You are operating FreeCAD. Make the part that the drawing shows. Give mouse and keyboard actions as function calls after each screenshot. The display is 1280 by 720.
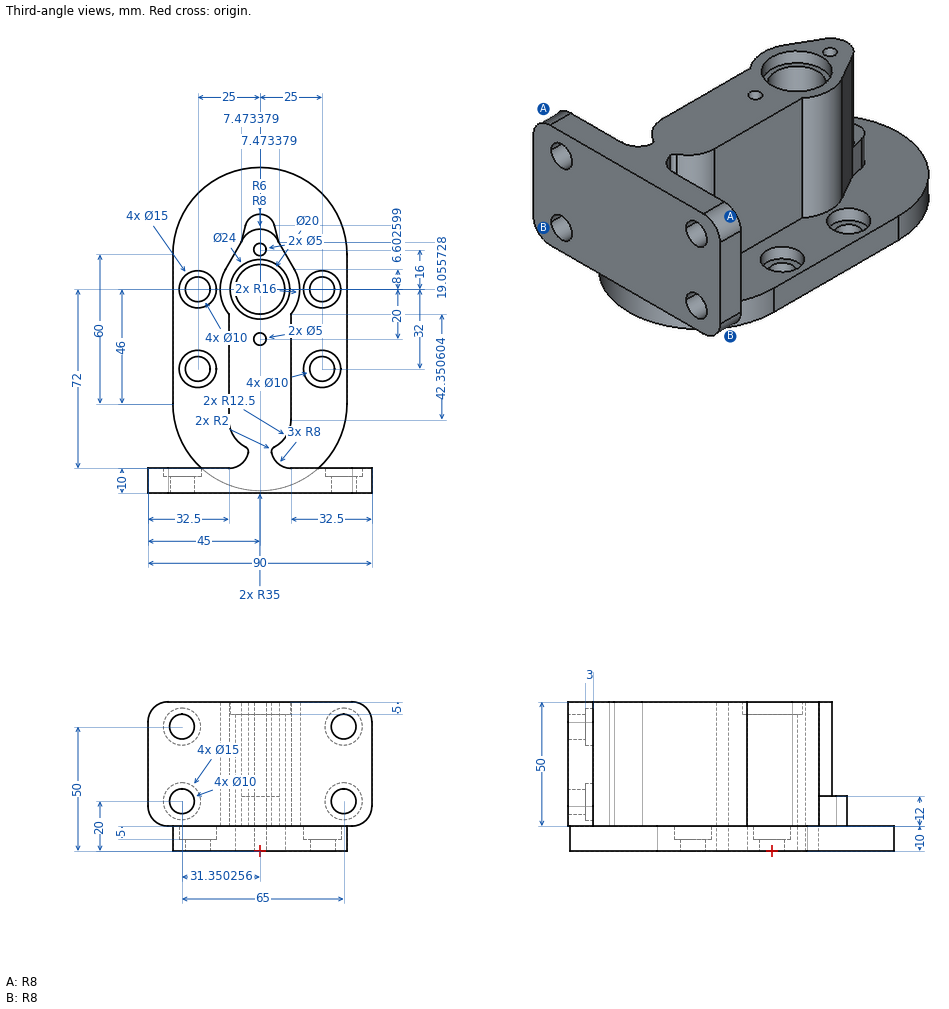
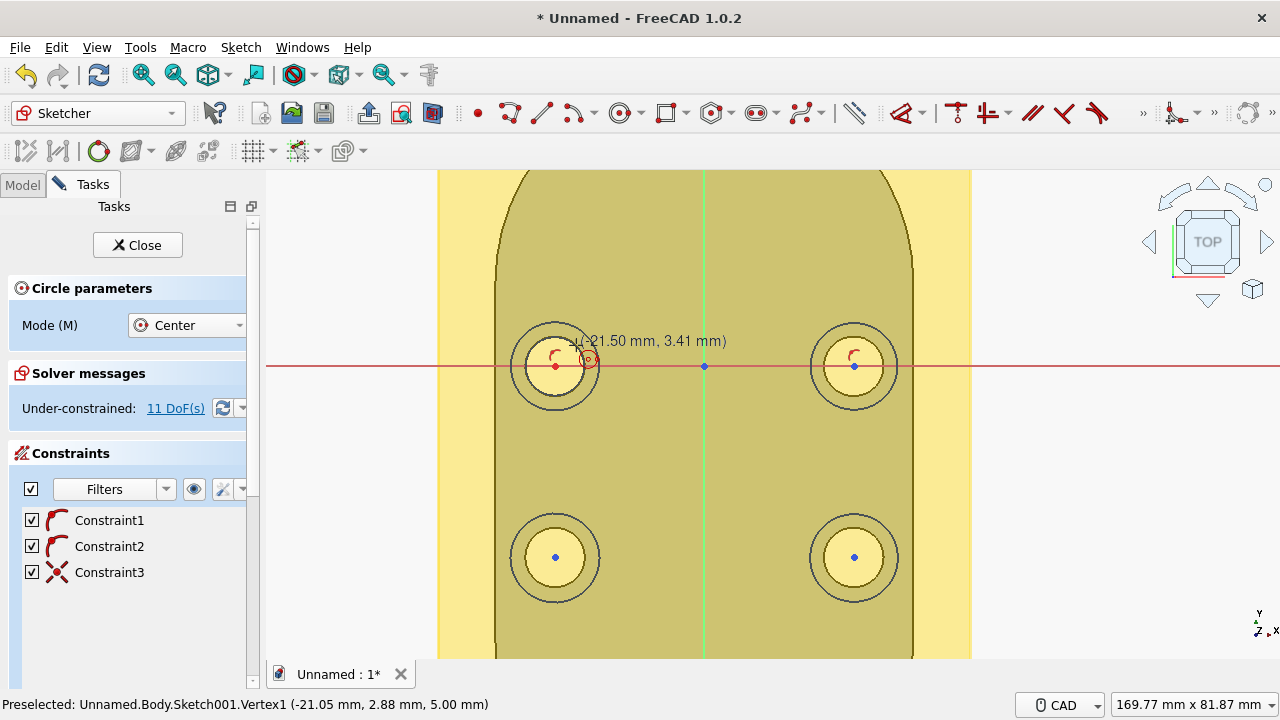
click(854, 366)
click(875, 345)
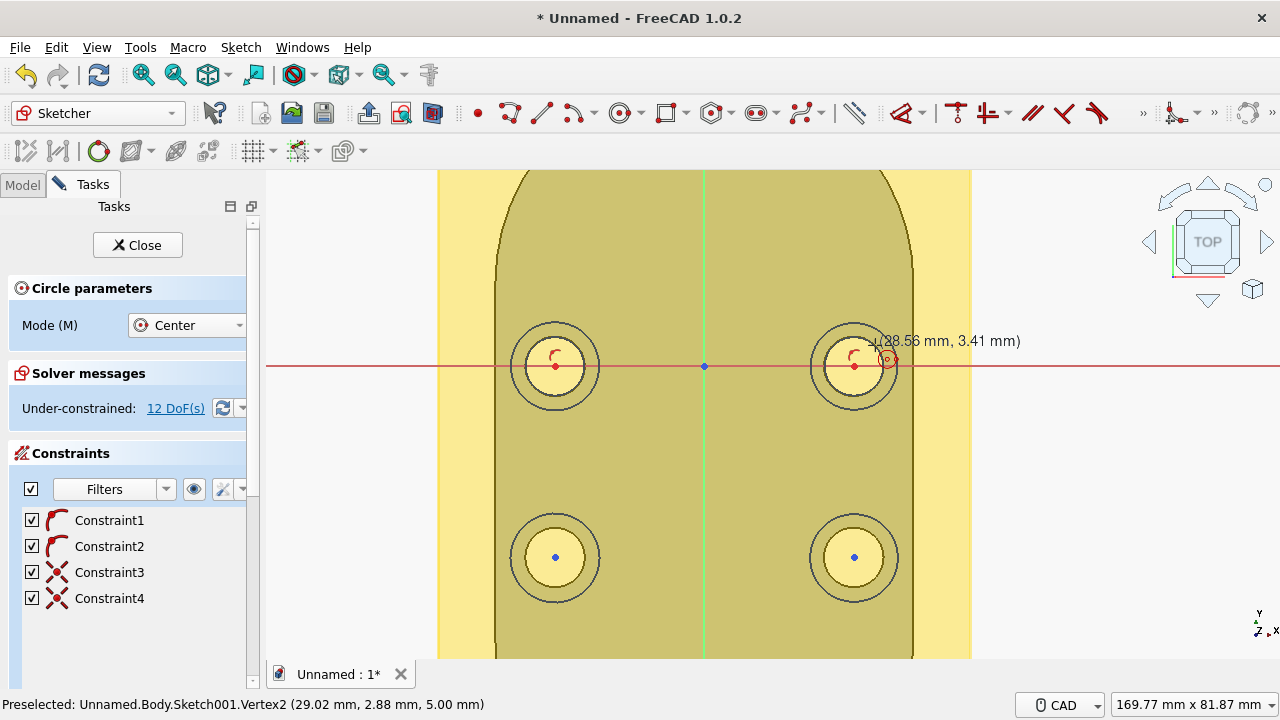
click(854, 558)
click(875, 536)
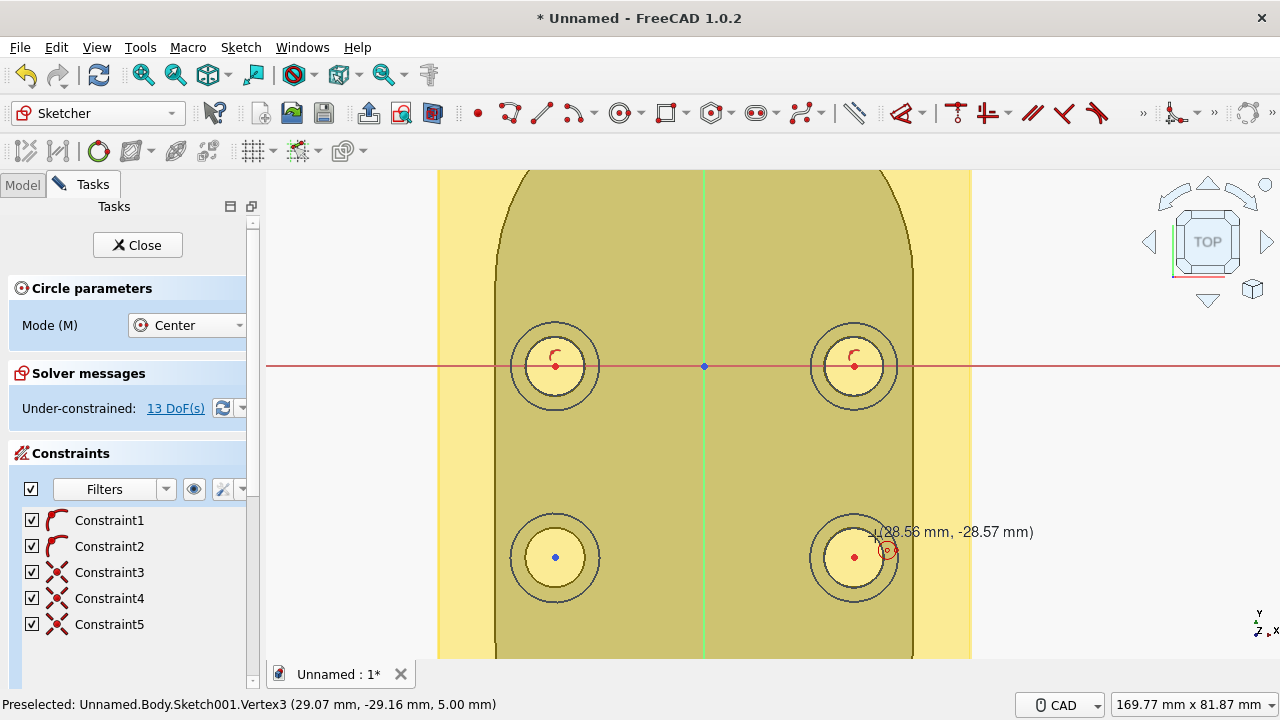
click(555, 558)
click(576, 536)
key(Escape)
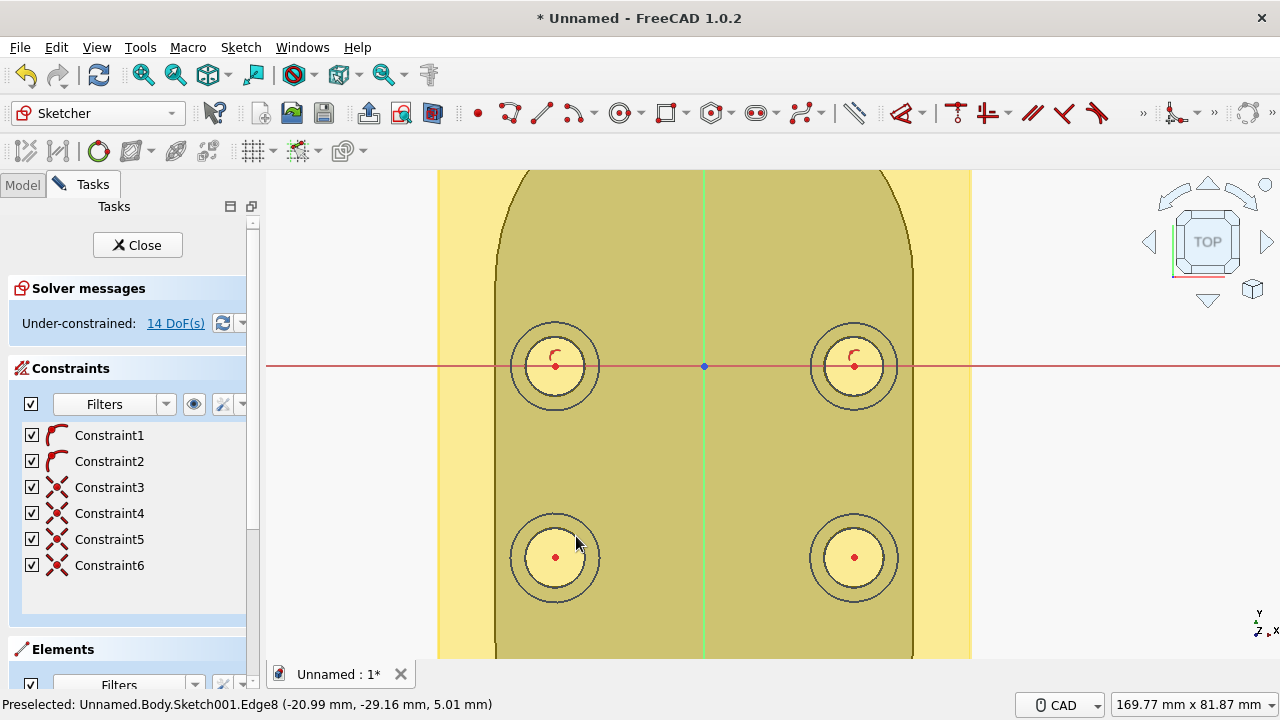
click(586, 335)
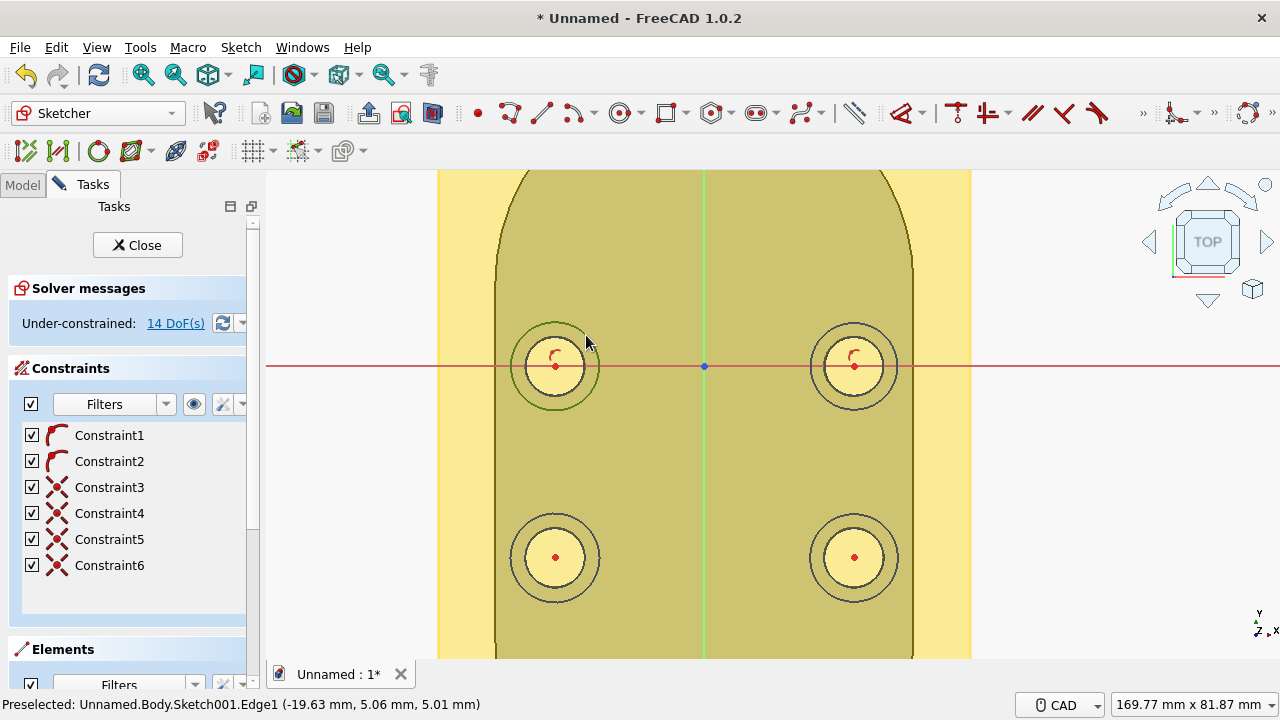
click(885, 336)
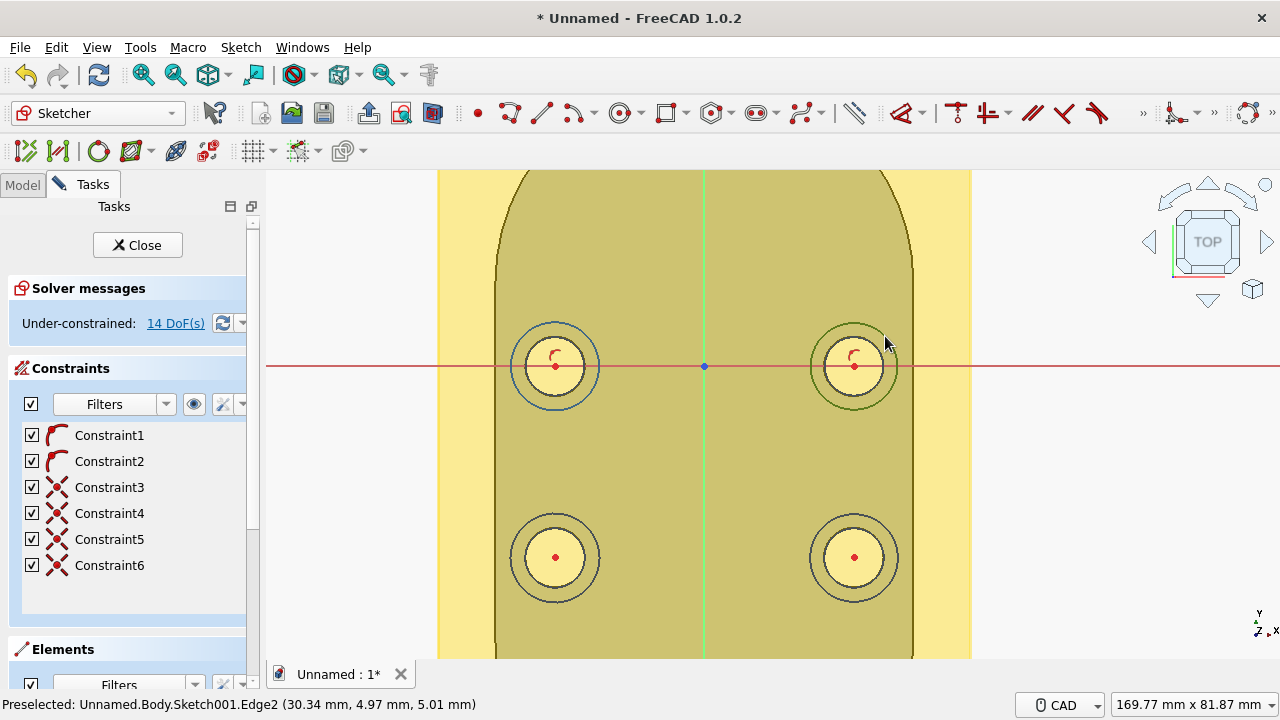
click(885, 527)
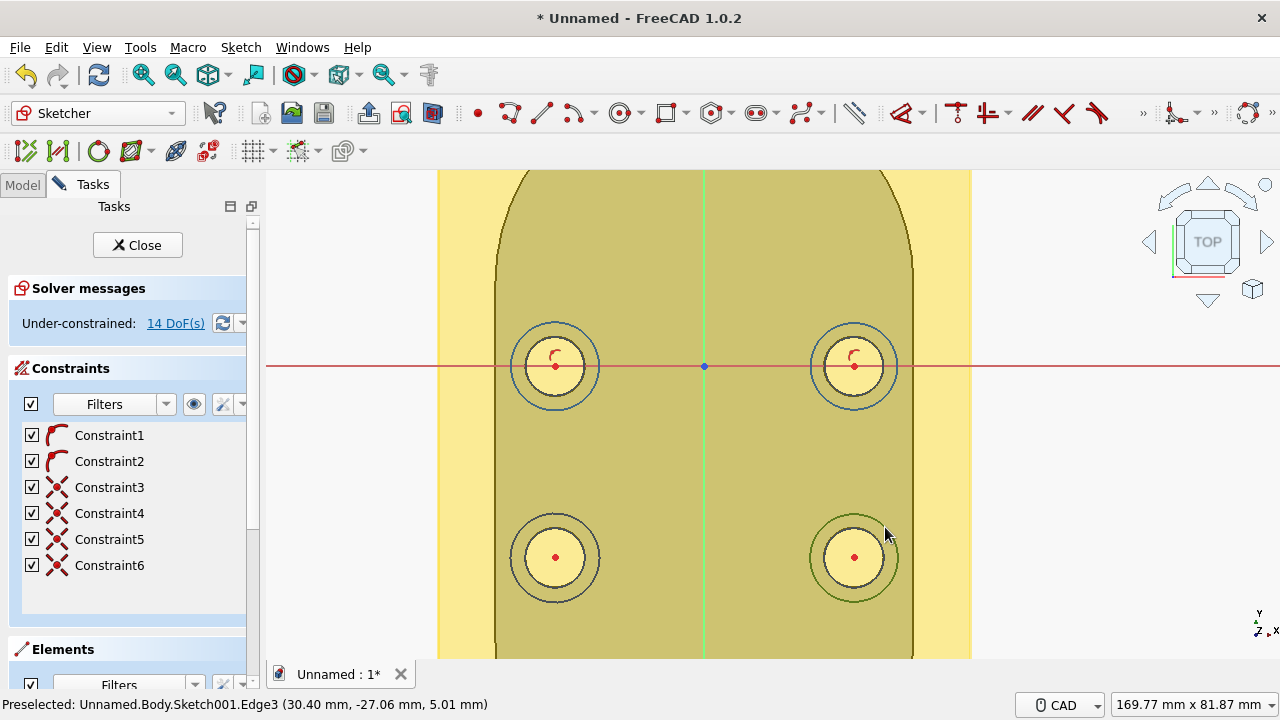
click(586, 526)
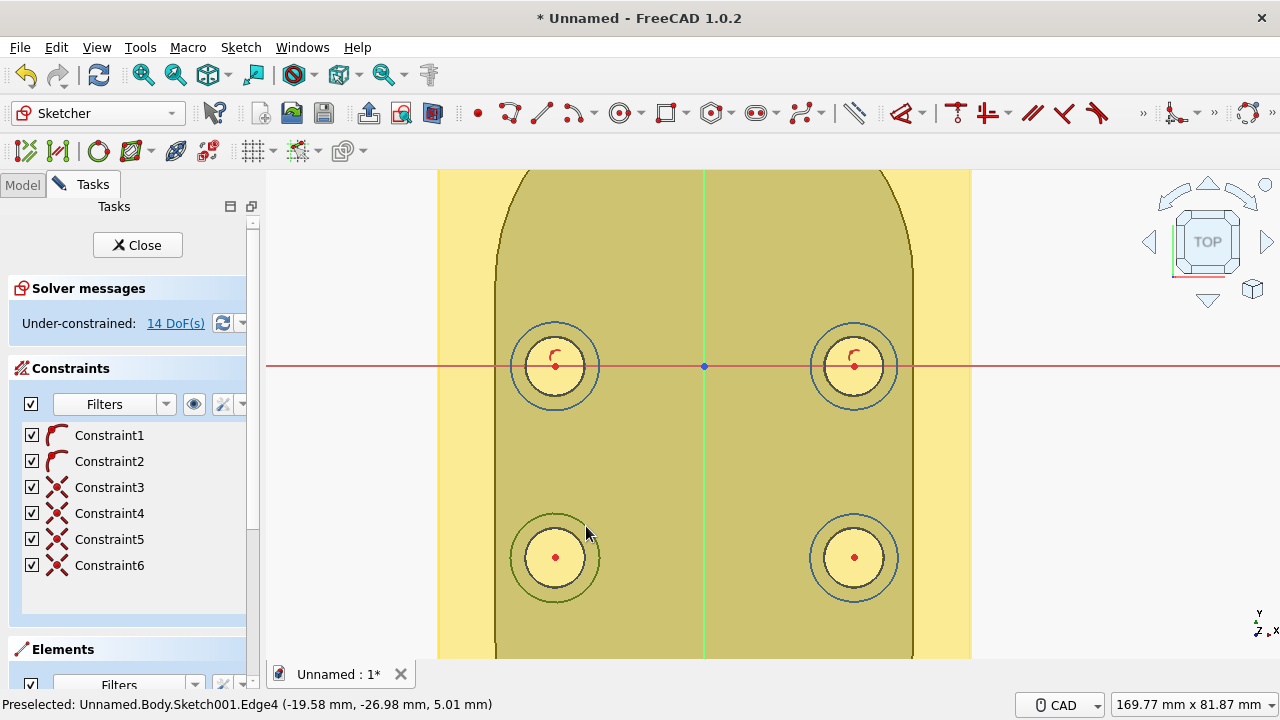
key(e)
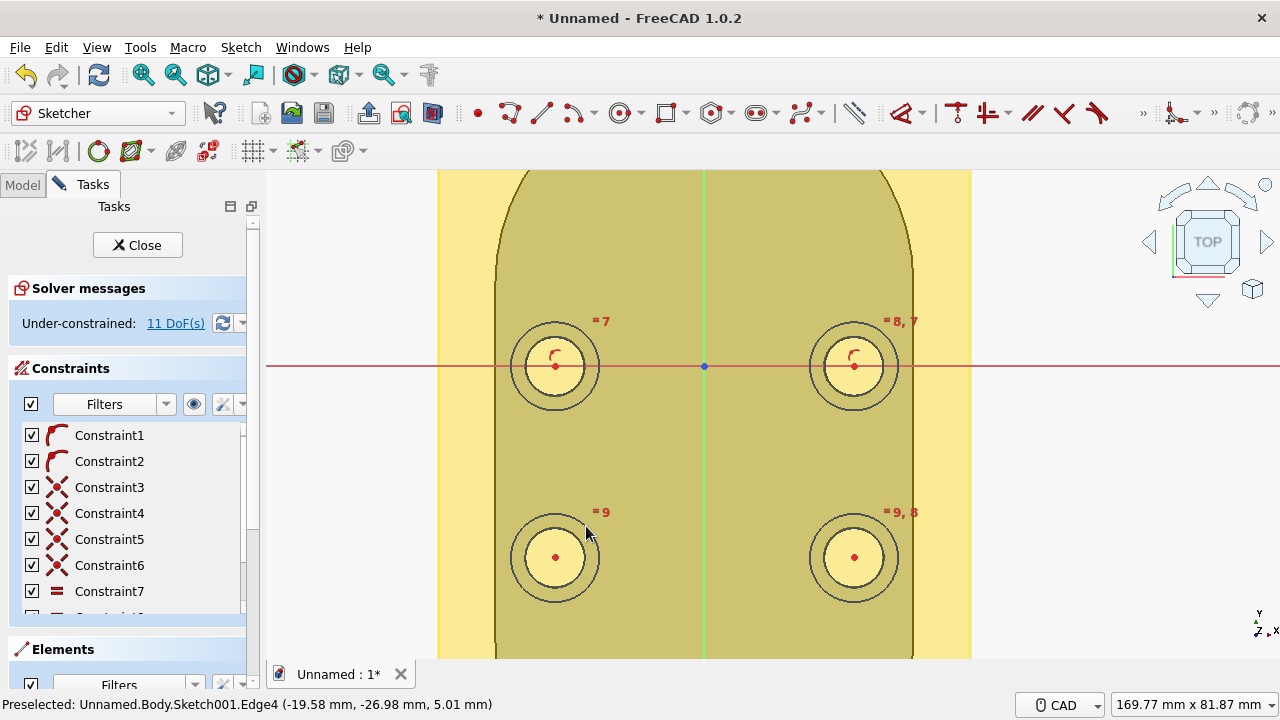
click(576, 346)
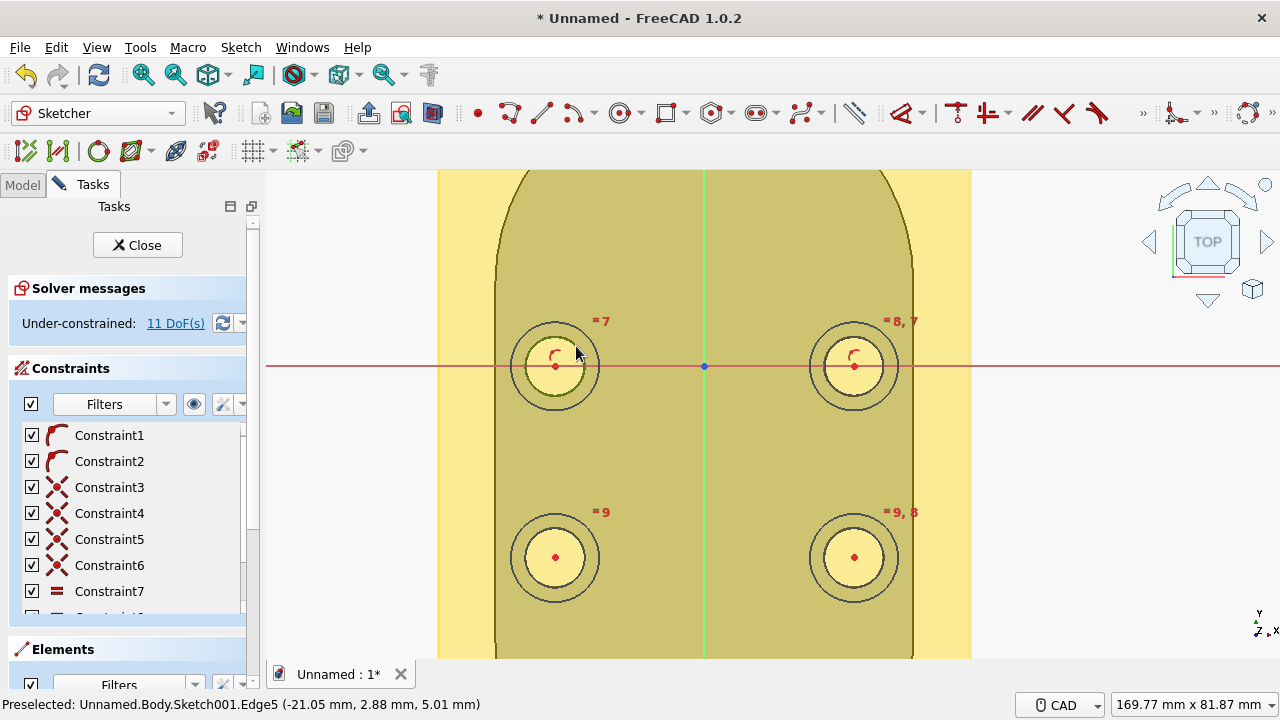
click(875, 346)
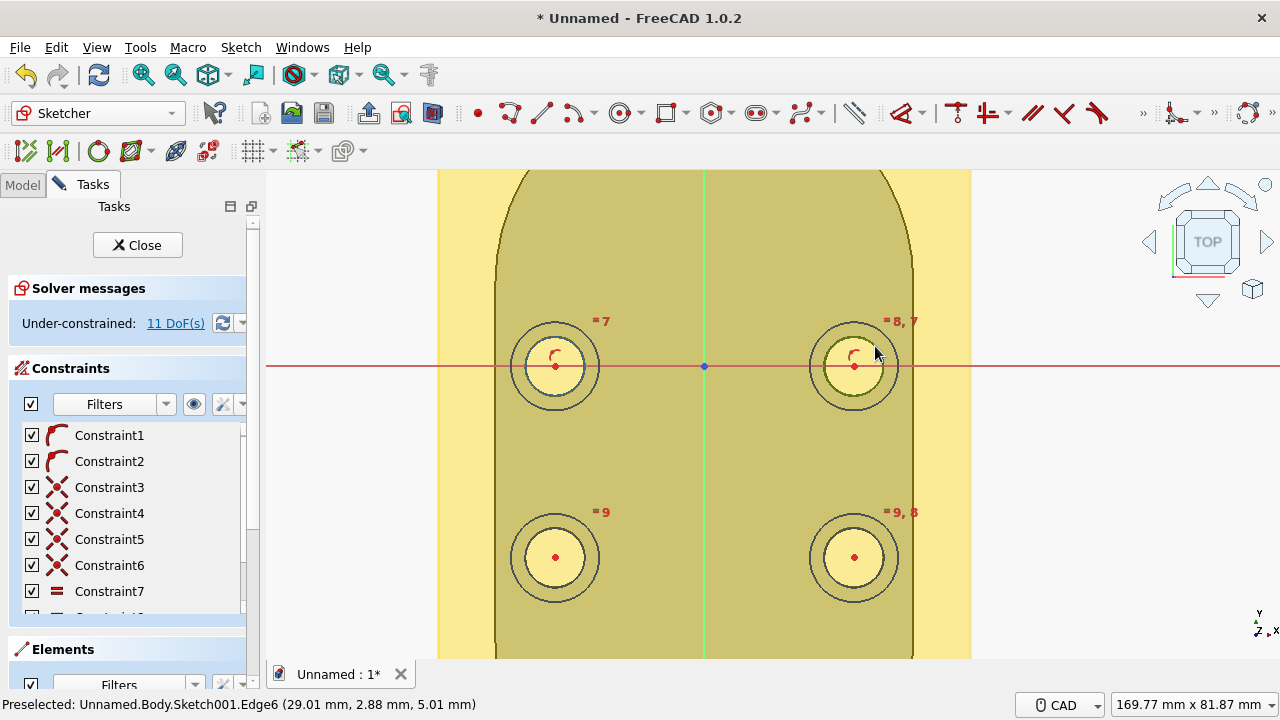
click(875, 537)